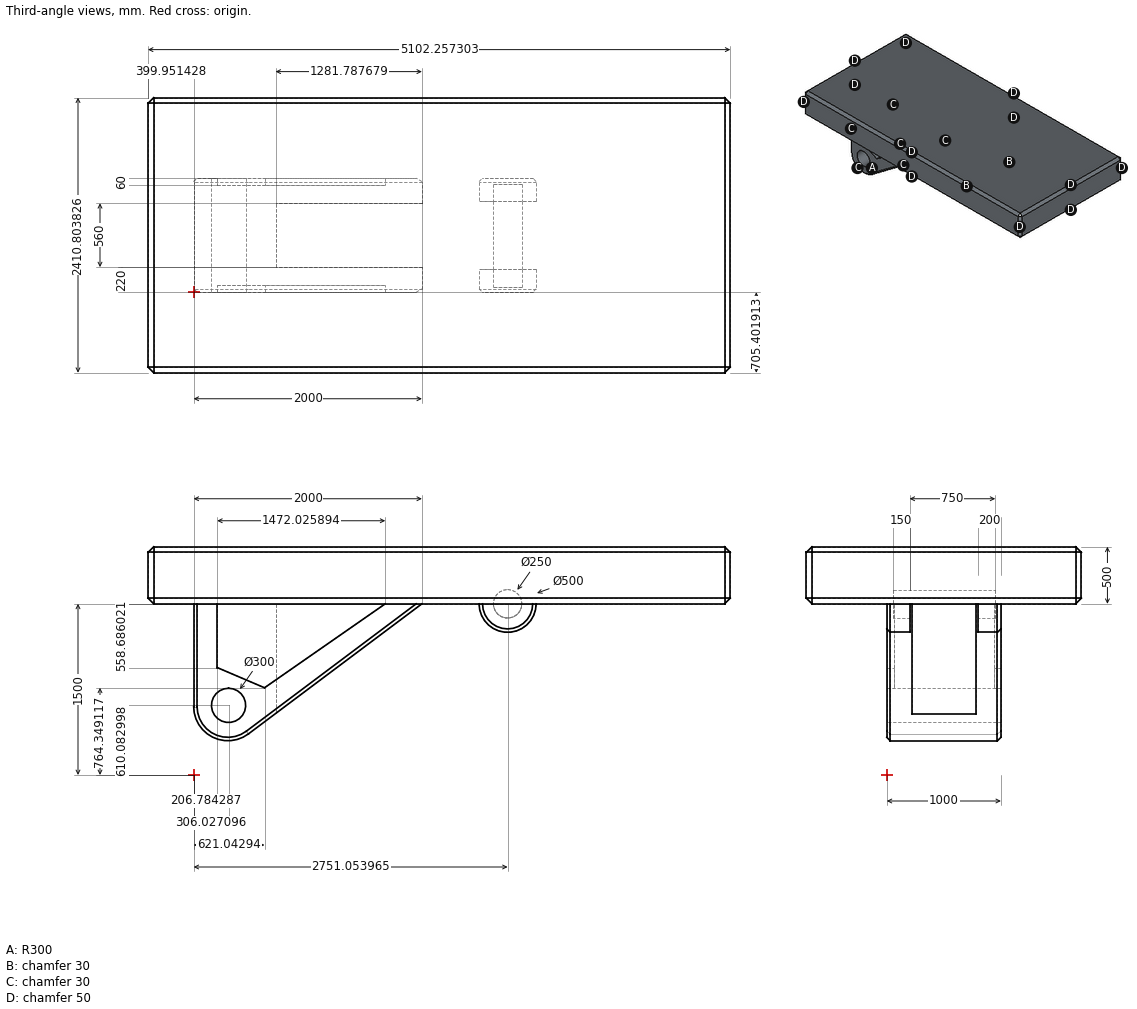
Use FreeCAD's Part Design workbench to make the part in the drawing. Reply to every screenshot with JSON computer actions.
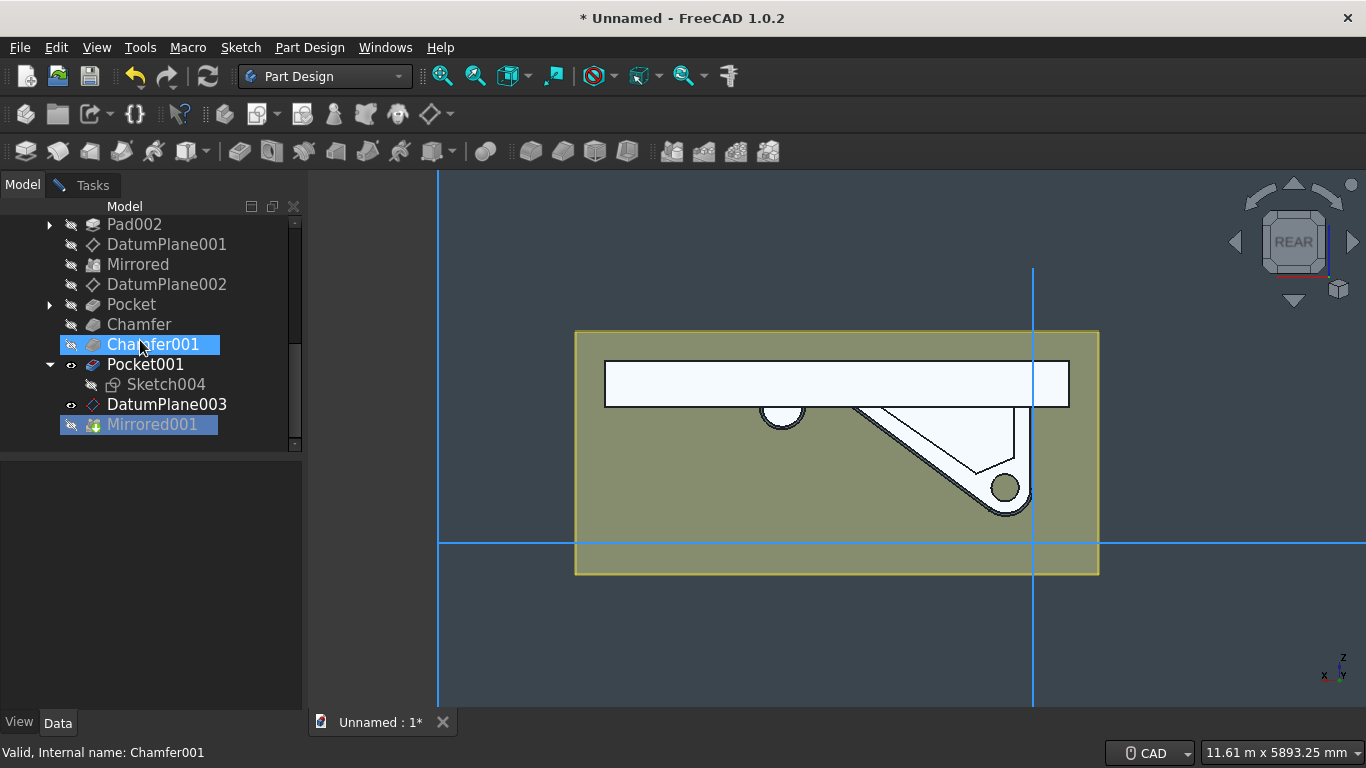
{"action": "left_click", "coordinate": [116, 405]}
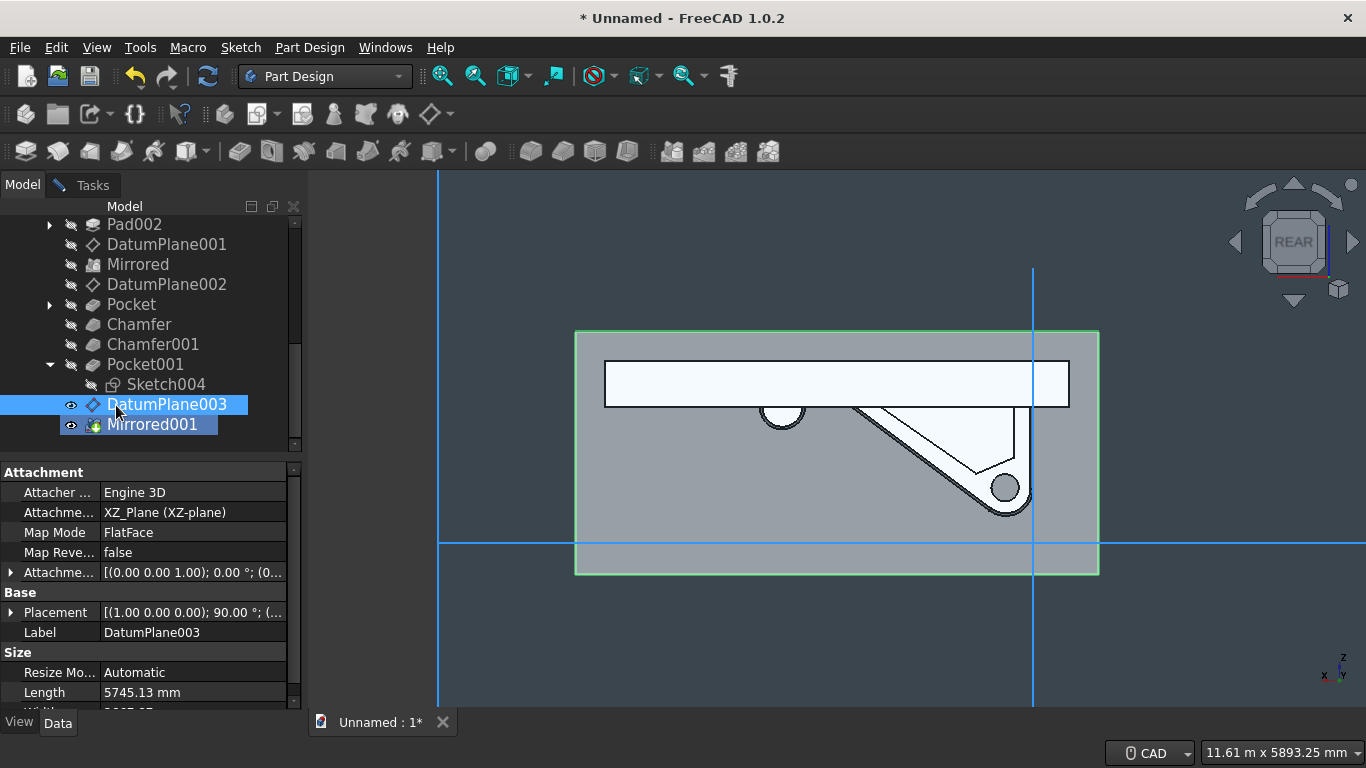
{"action": "left_click", "coordinate": [84, 184]}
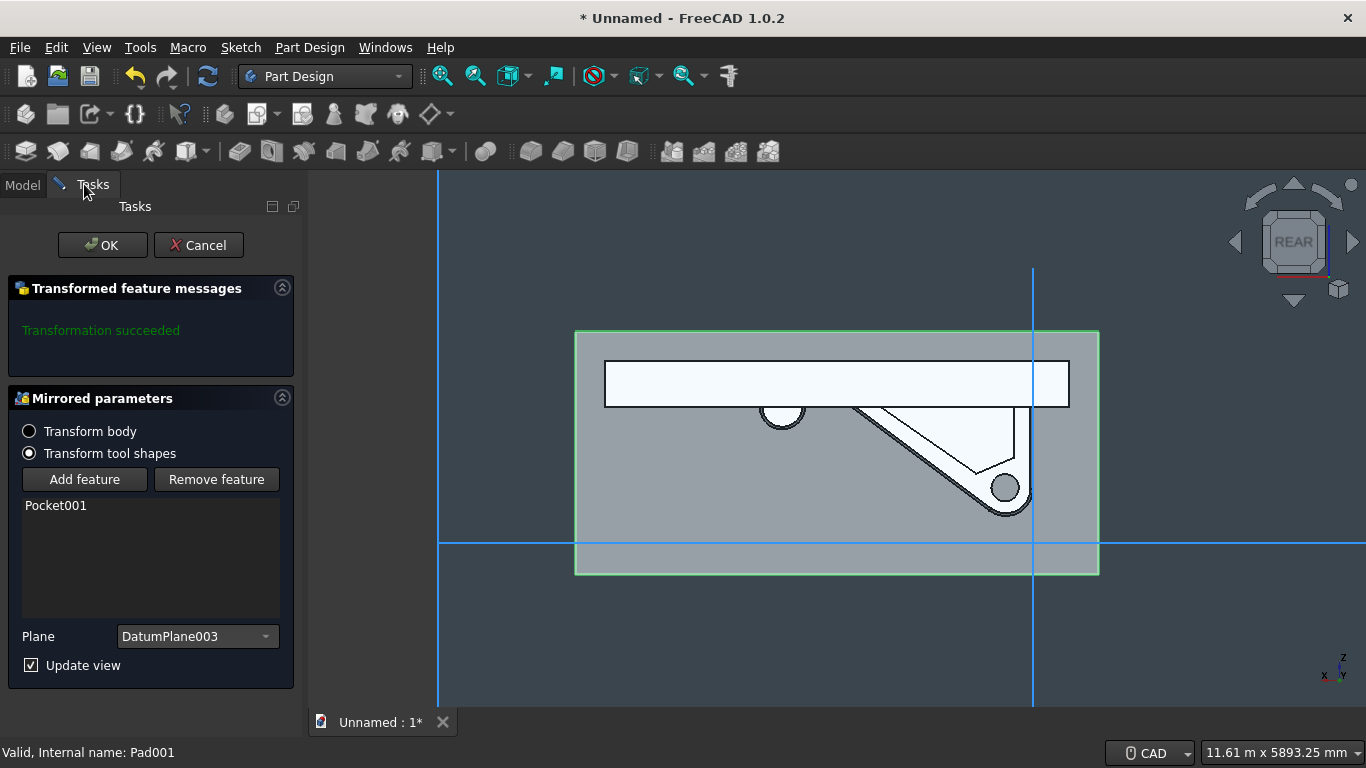
{"action": "left_click", "coordinate": [103, 245]}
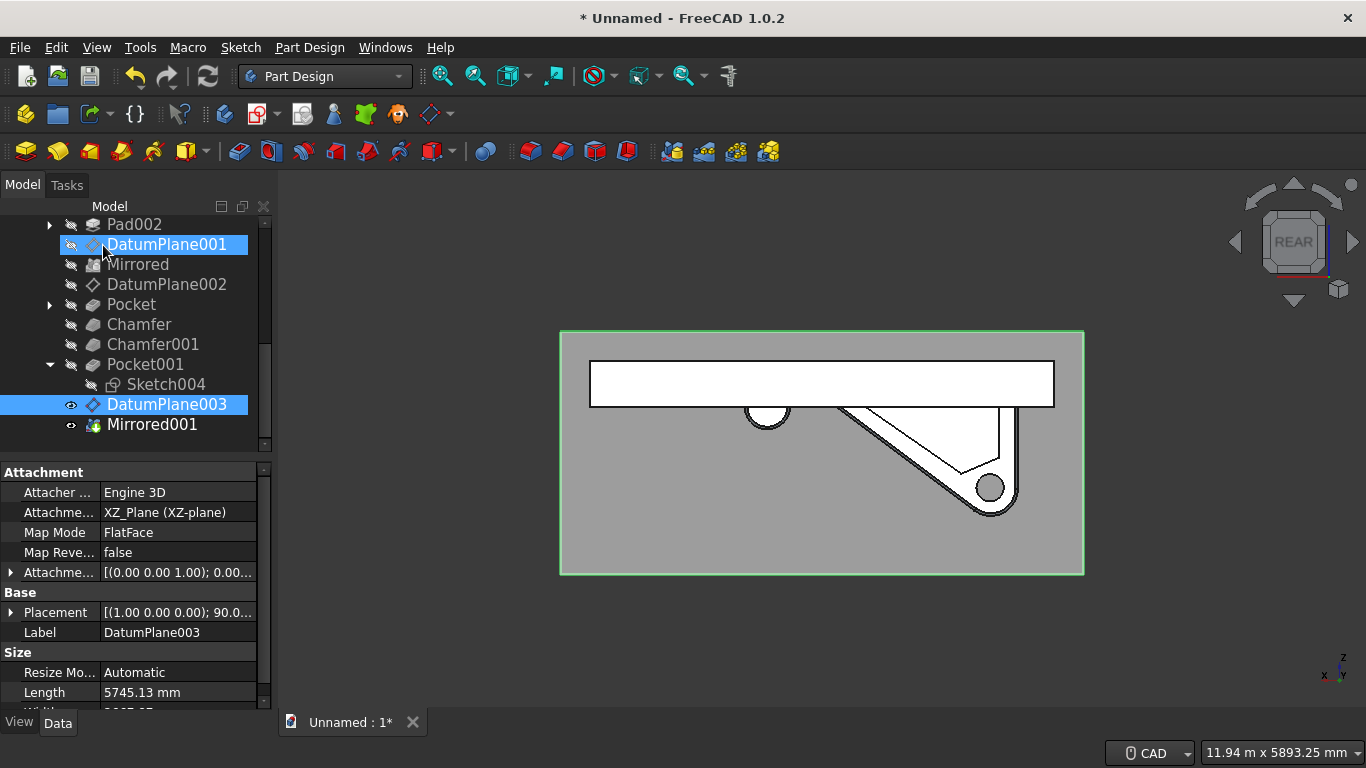
{"action": "left_click", "coordinate": [116, 405]}
{"action": "key", "text": "space"}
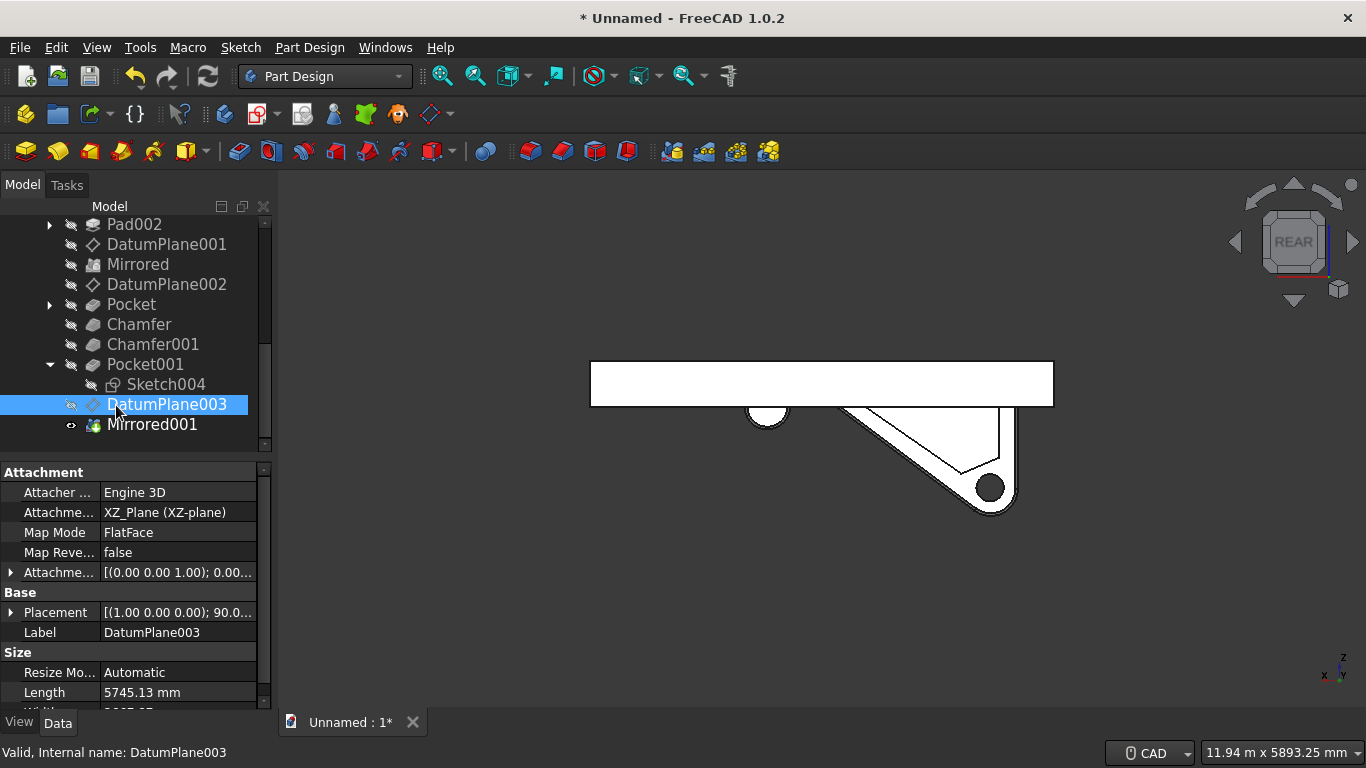
{"action": "left_click", "coordinate": [444, 76]}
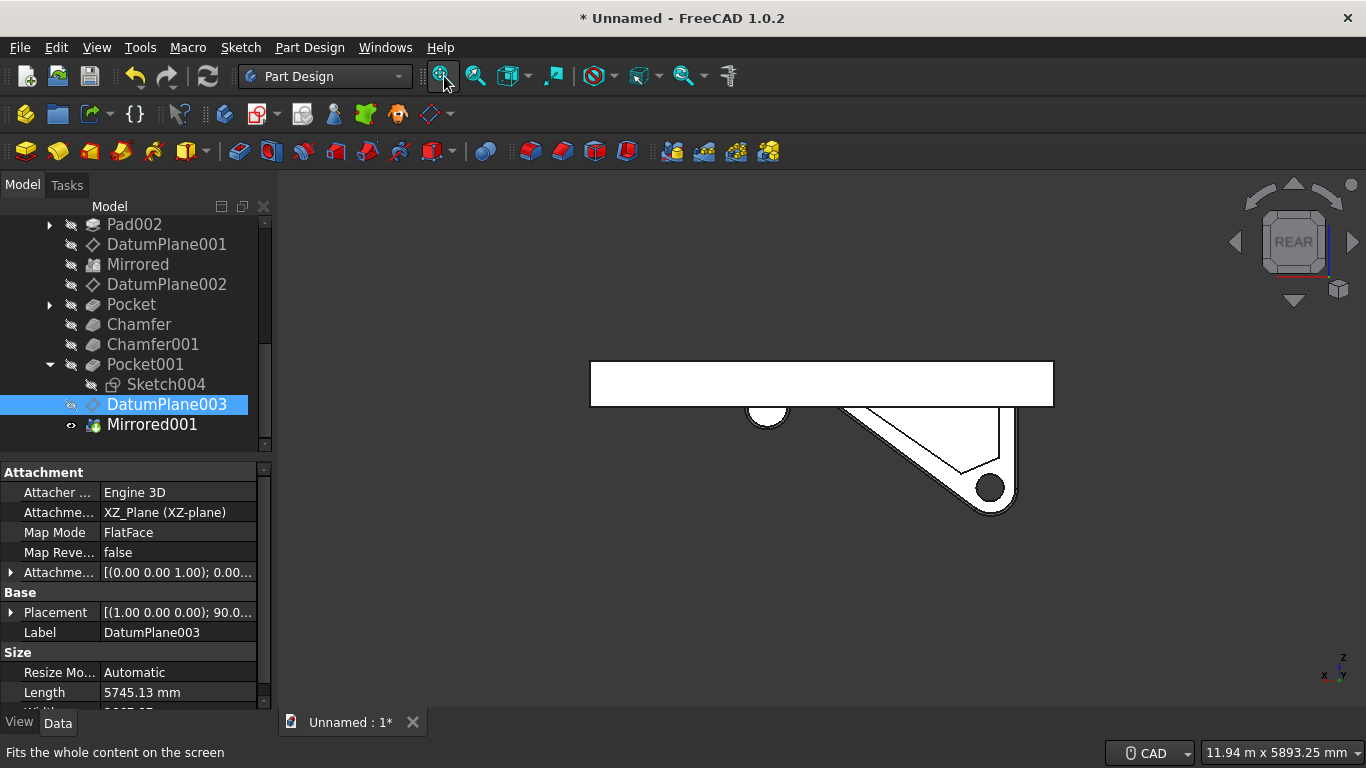
{"action": "left_click", "coordinate": [623, 383]}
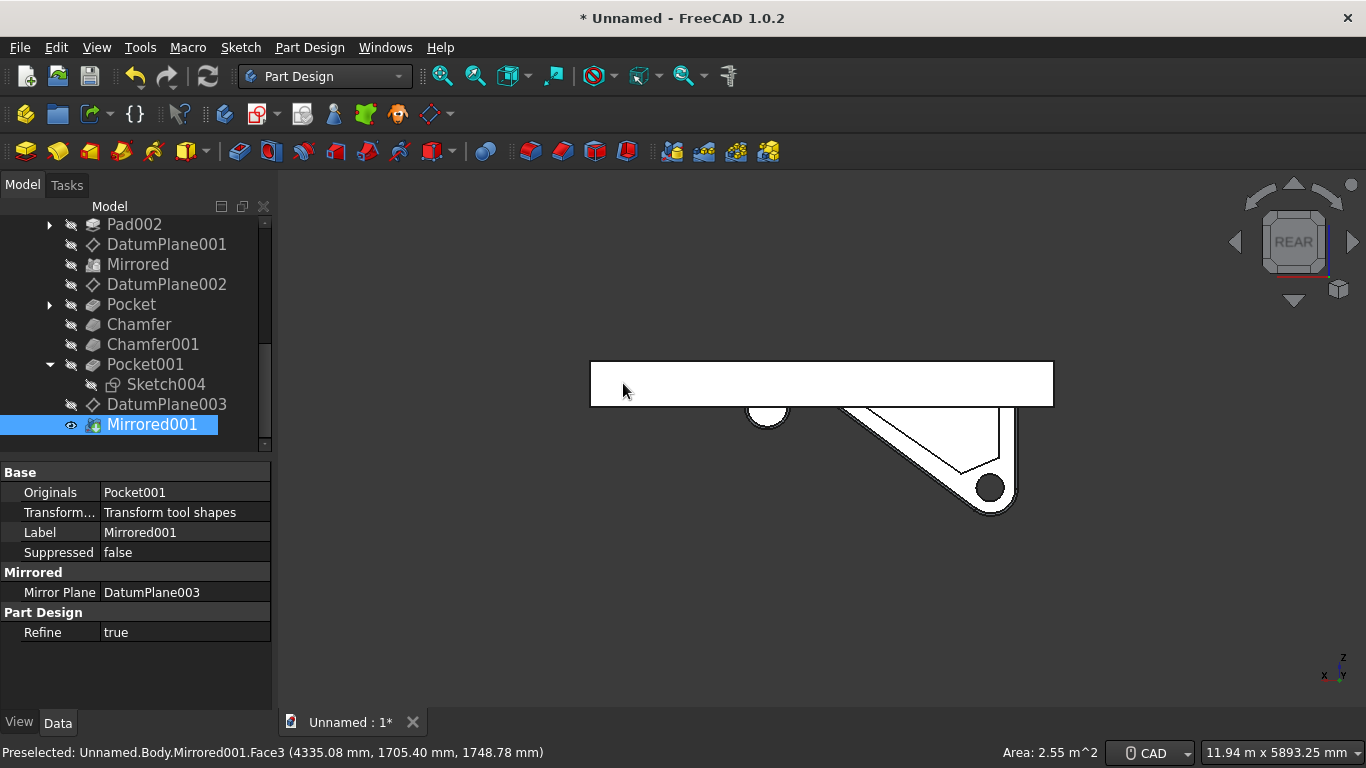
{"action": "key", "text": "0"}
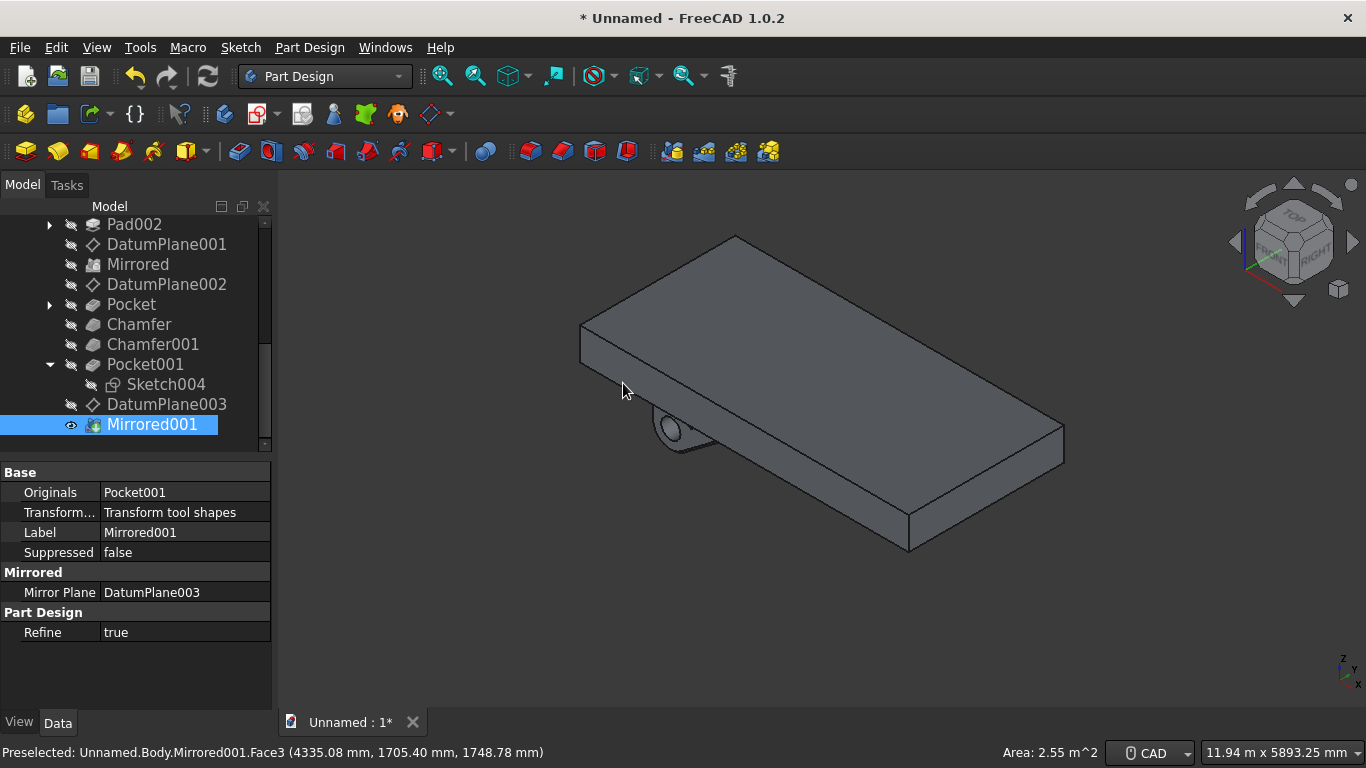
{"action": "left_click", "coordinate": [869, 401], "text": "ctrl"}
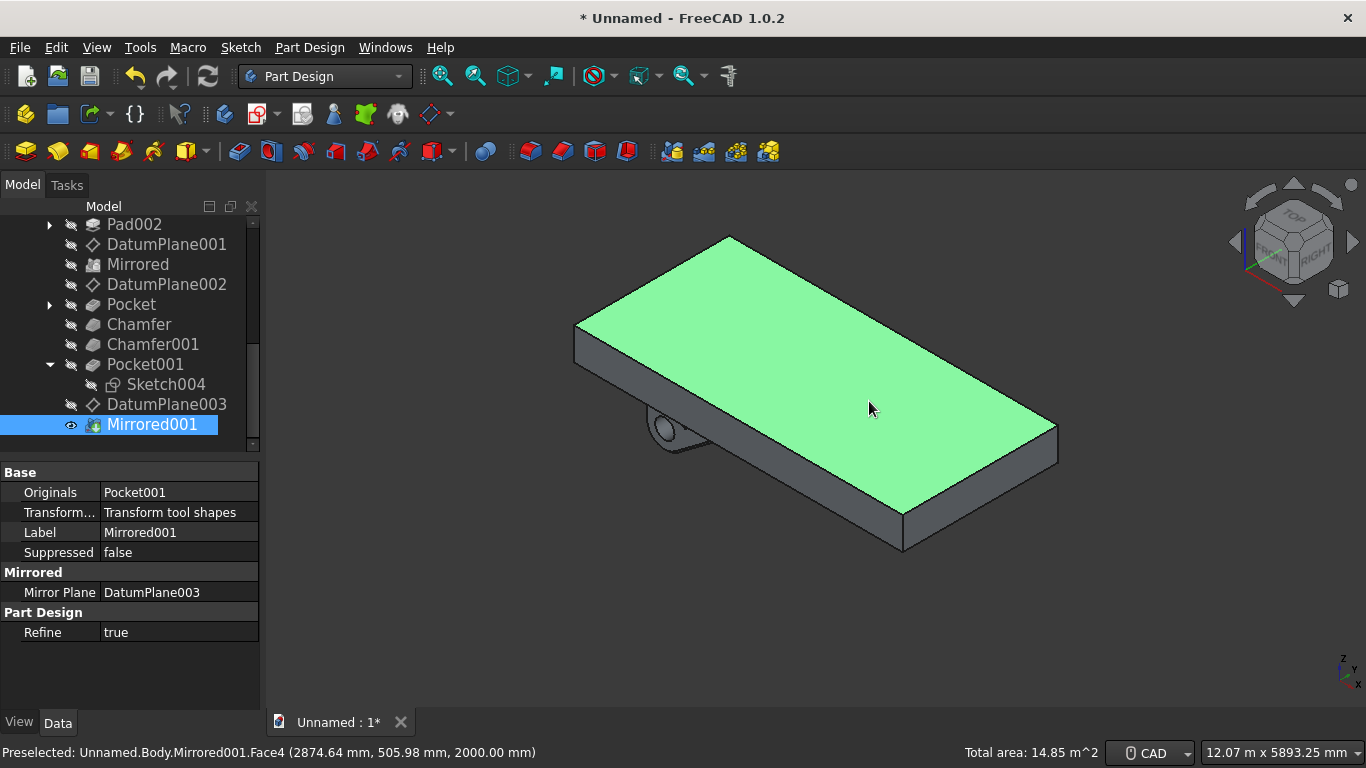
{"action": "left_click", "coordinate": [879, 519], "text": "ctrl"}